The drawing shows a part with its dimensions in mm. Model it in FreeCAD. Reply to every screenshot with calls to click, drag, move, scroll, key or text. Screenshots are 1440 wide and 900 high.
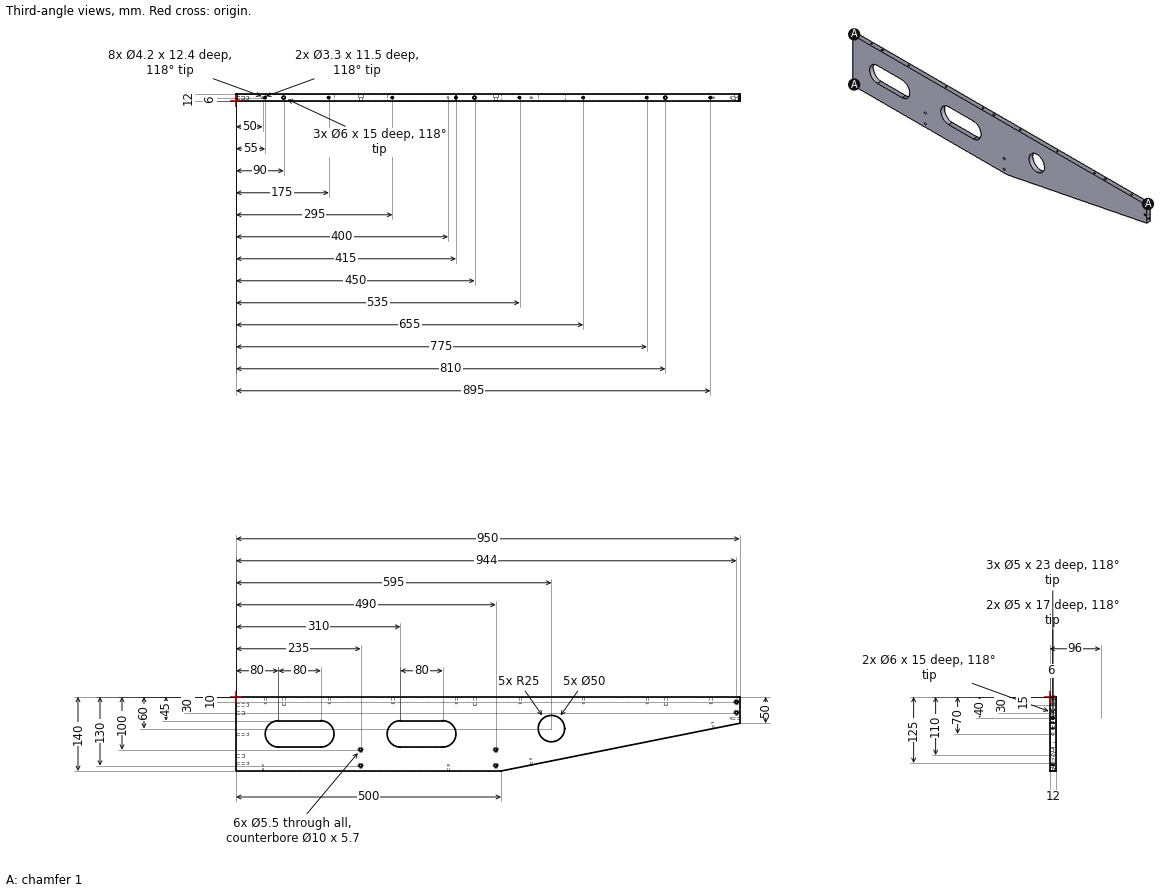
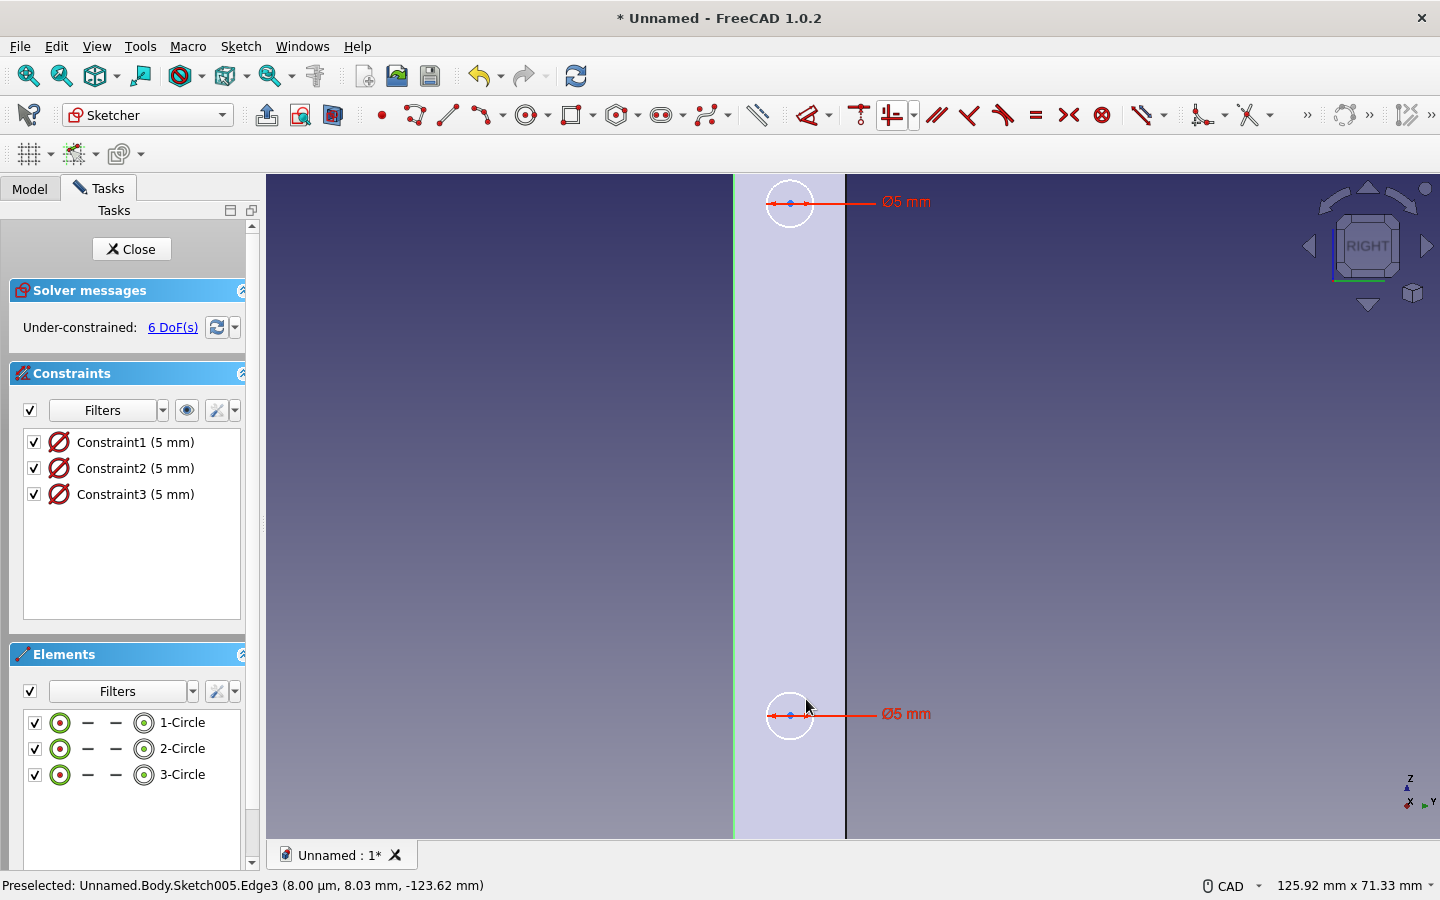
click(806, 116)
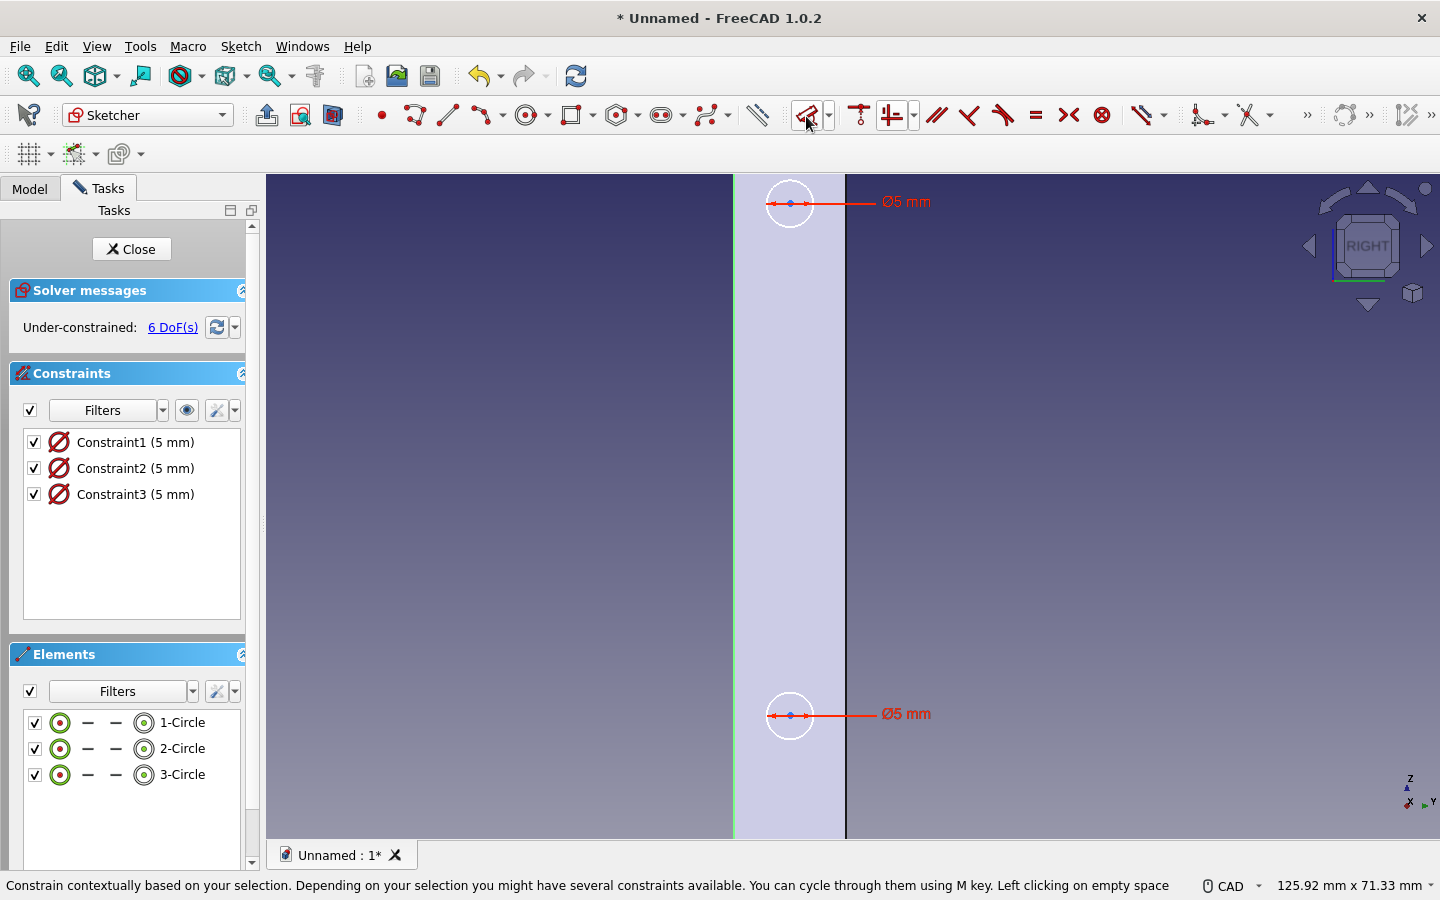
scroll(791, 717, down, 5)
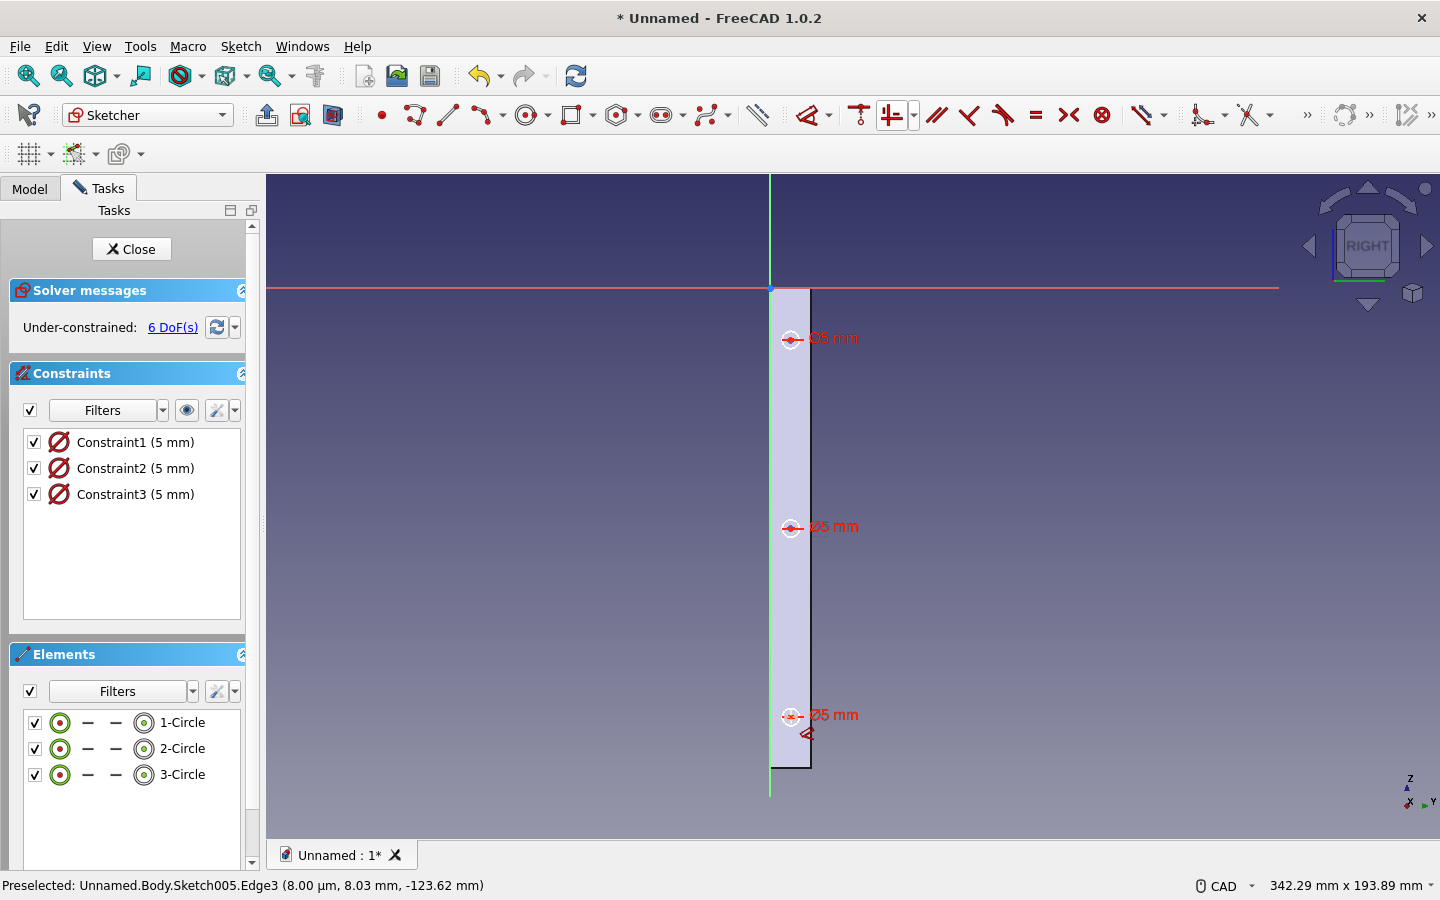
scroll(791, 340, up, 4)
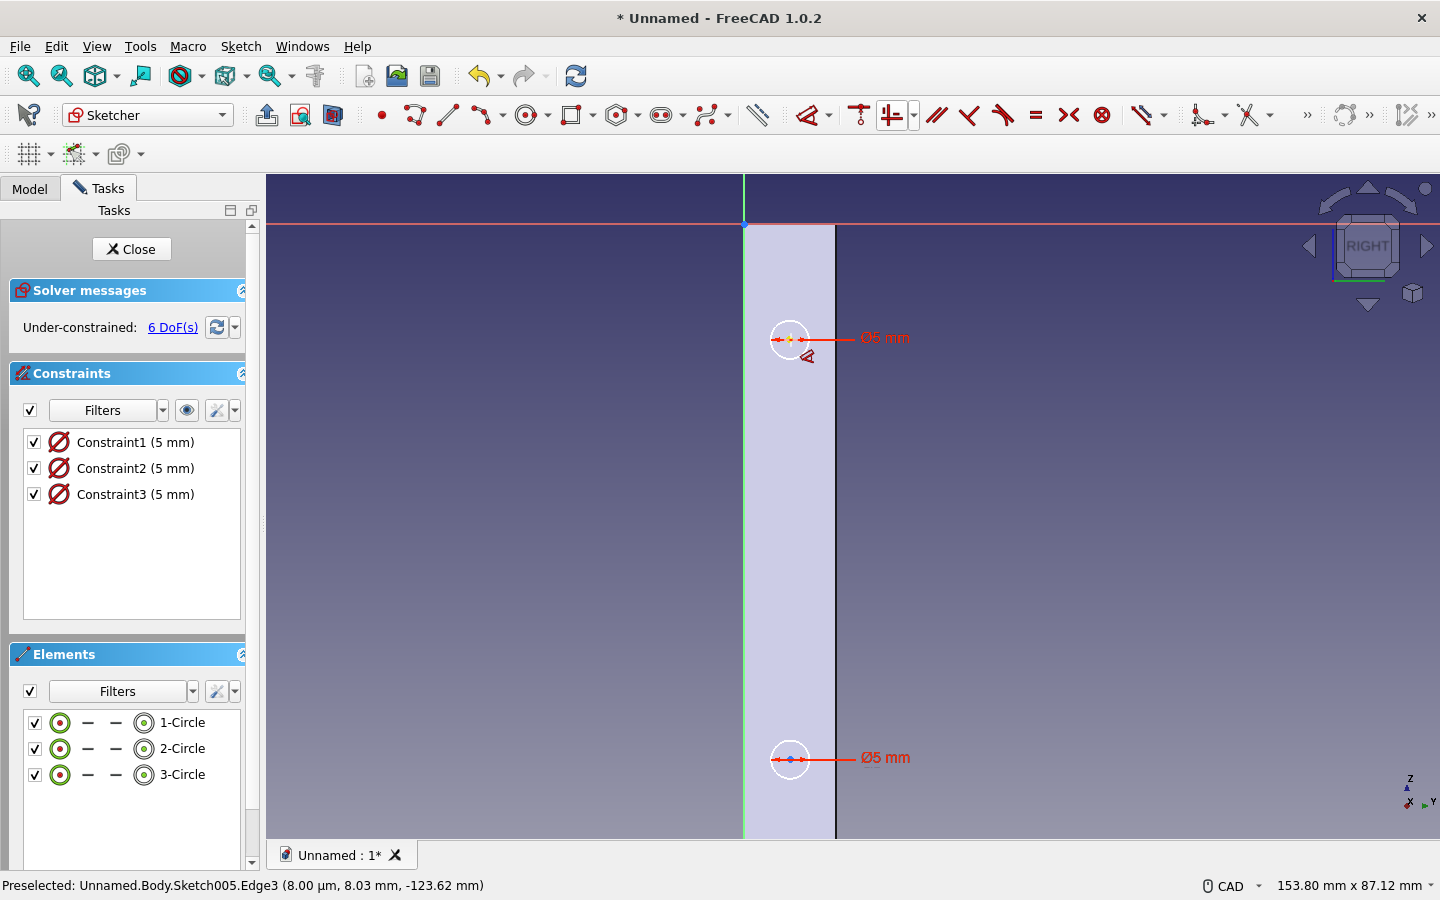
click(790, 340)
click(767, 374)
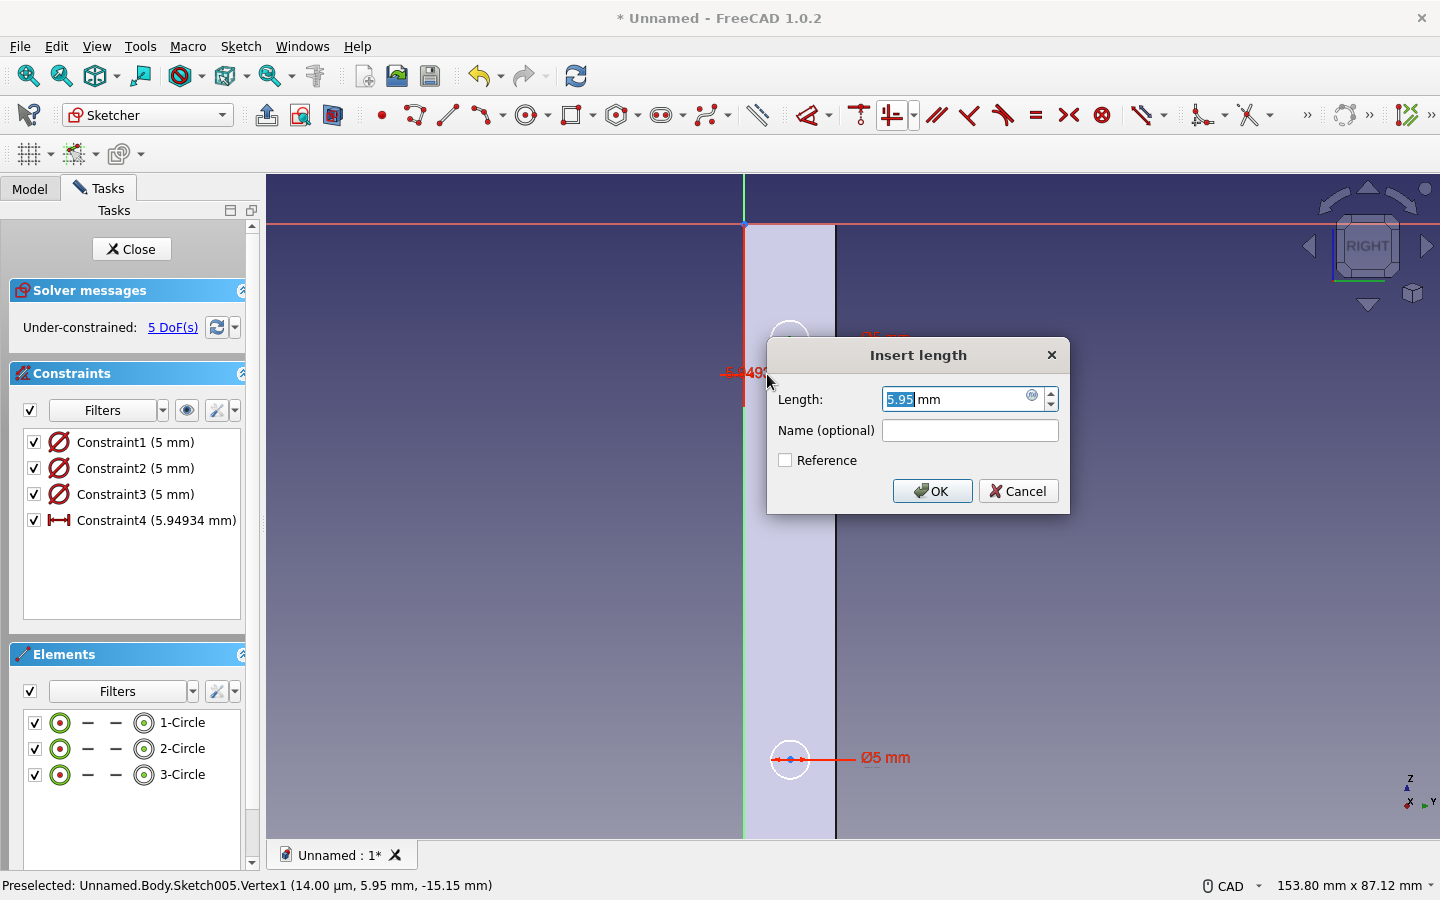
text(6)
key(Return)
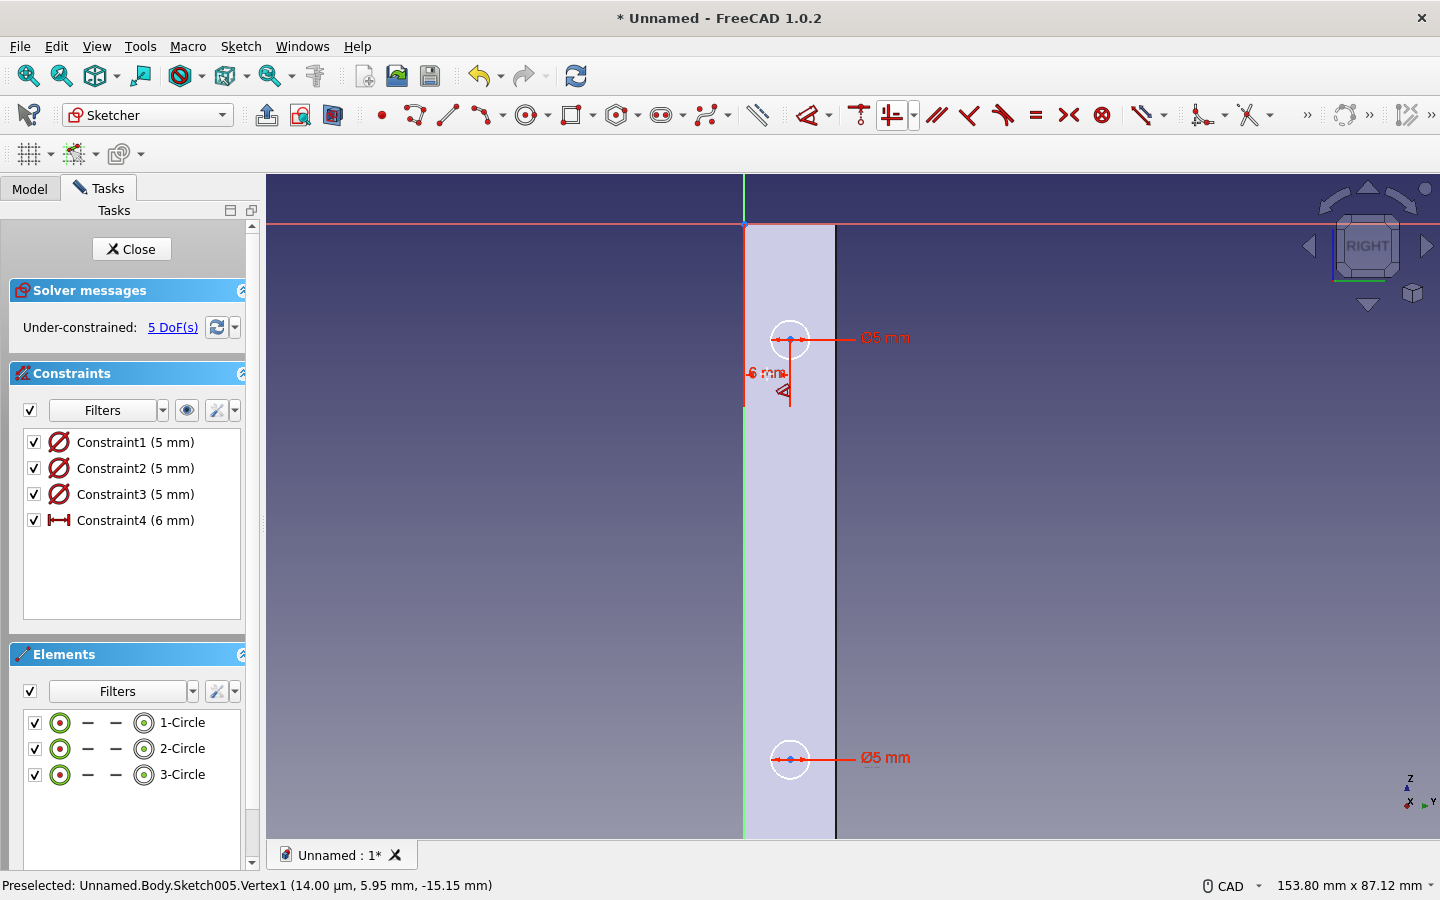
click(790, 760)
click(767, 794)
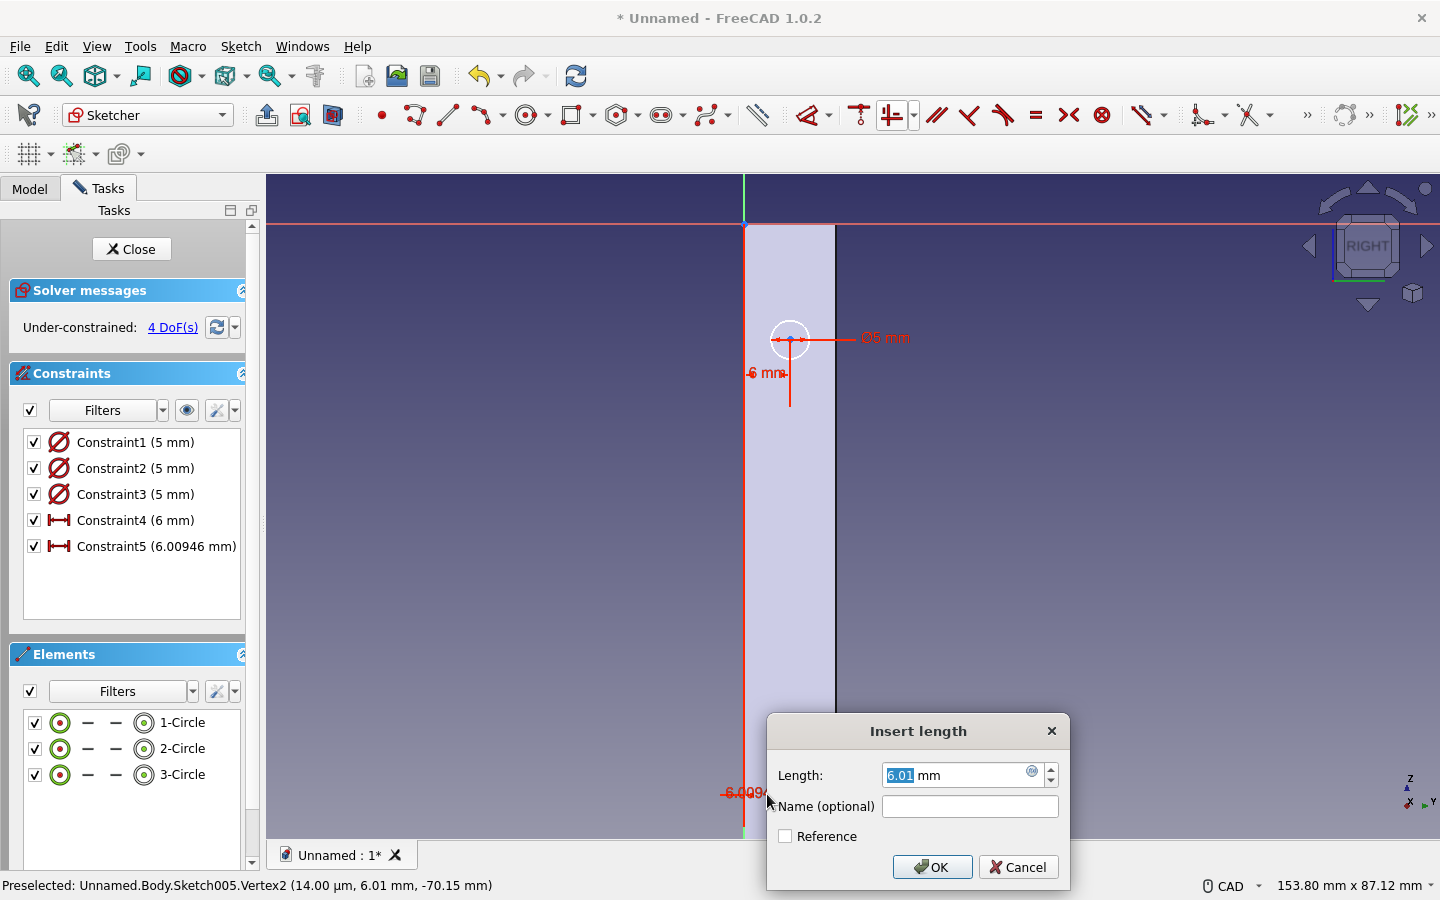
text(6)
key(Return)